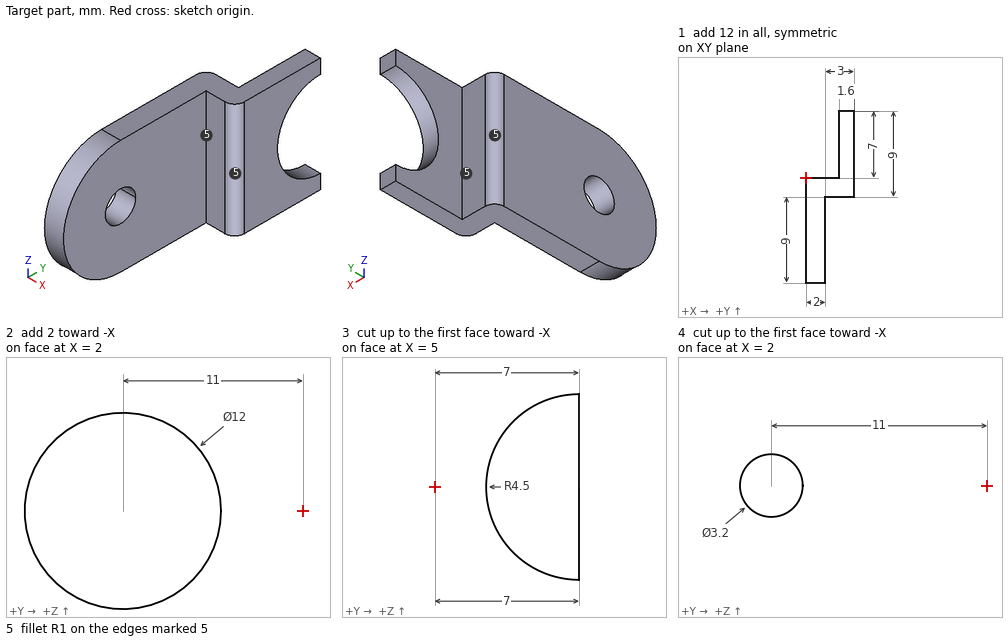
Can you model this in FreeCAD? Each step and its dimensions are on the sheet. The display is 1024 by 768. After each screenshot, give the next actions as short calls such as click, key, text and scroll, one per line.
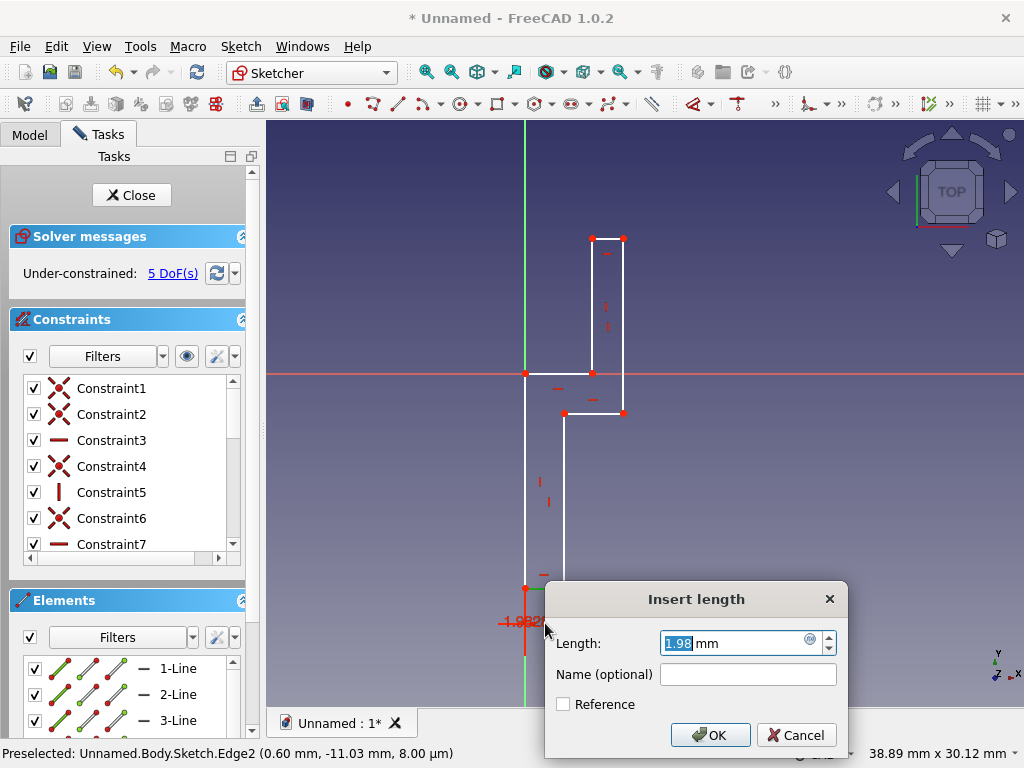
text(2)
key(Return)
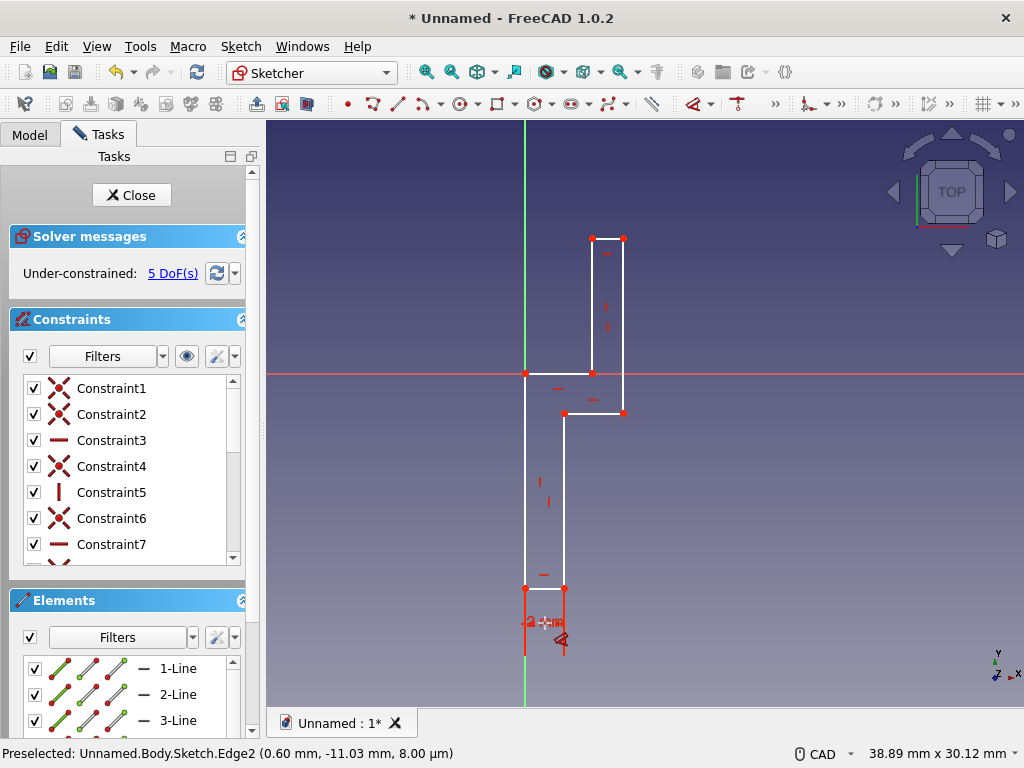
click(564, 536)
click(598, 501)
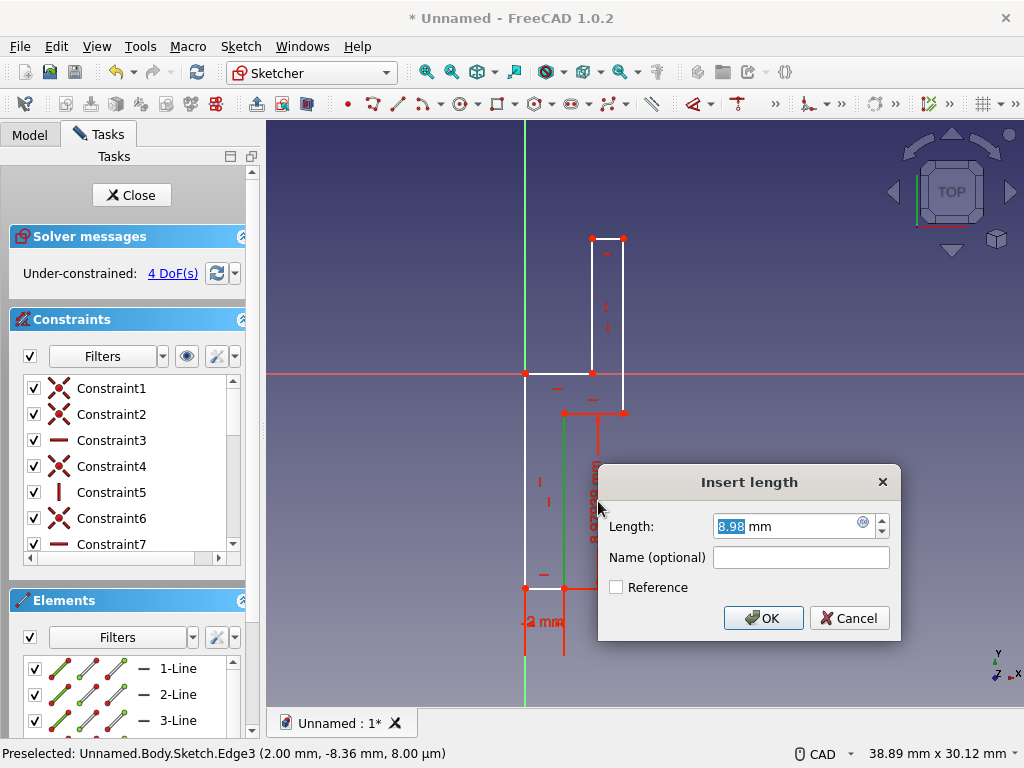
text(9)
key(Return)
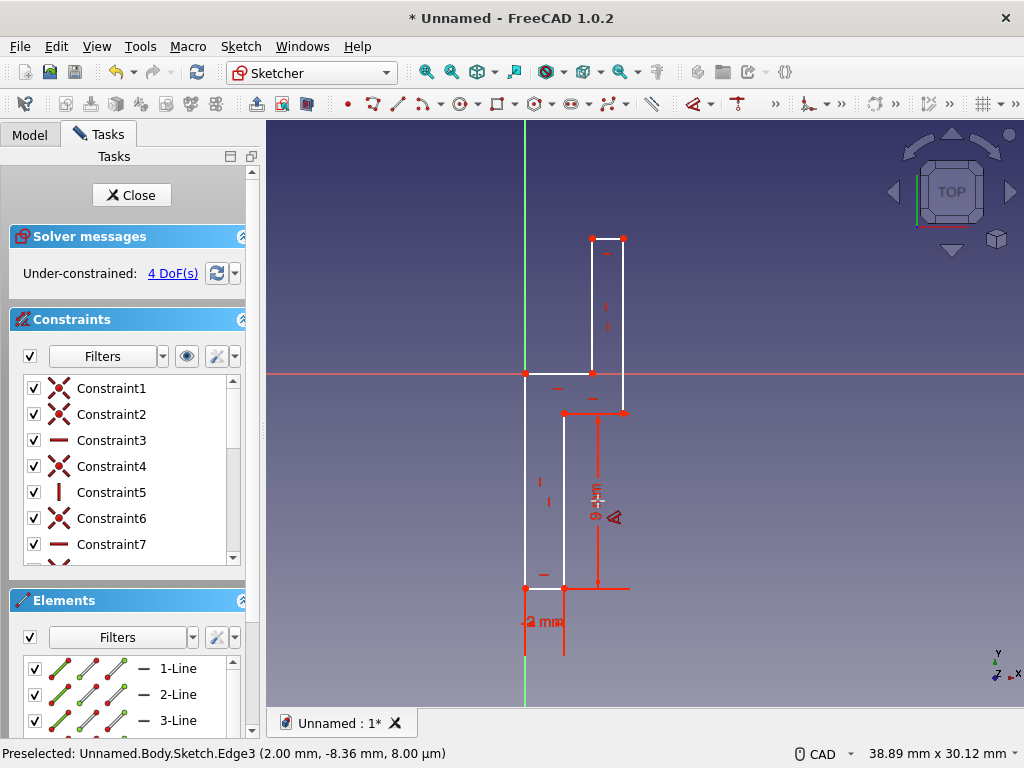
click(582, 414)
click(594, 448)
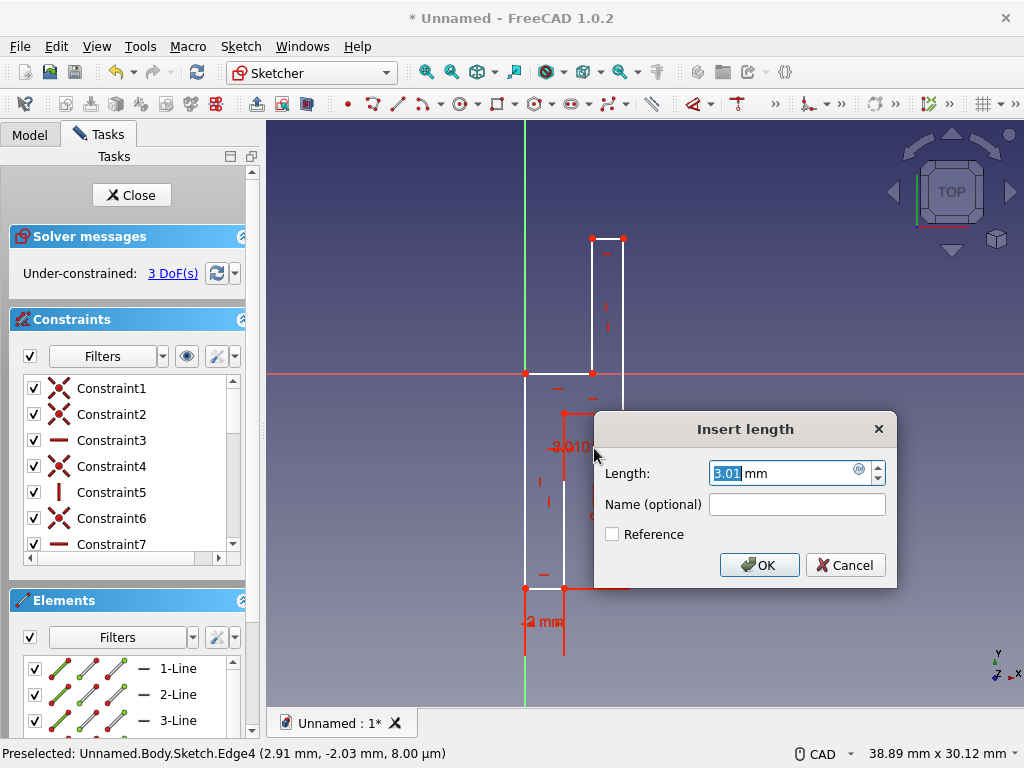
text(3)
key(Return)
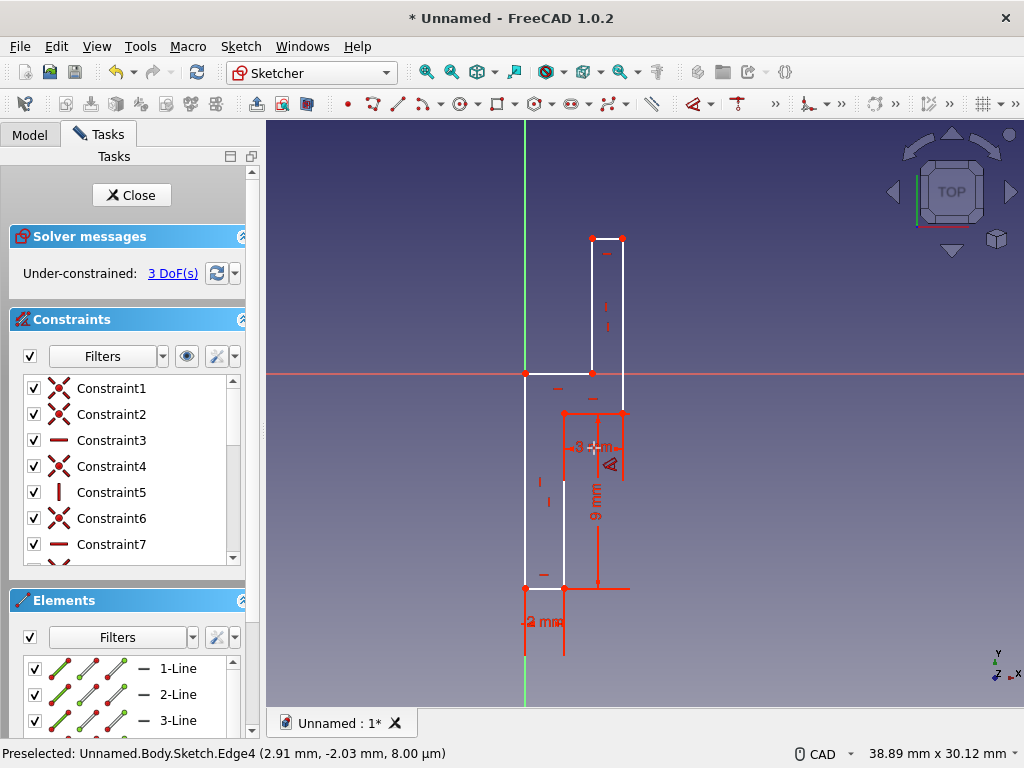
click(623, 361)
click(657, 326)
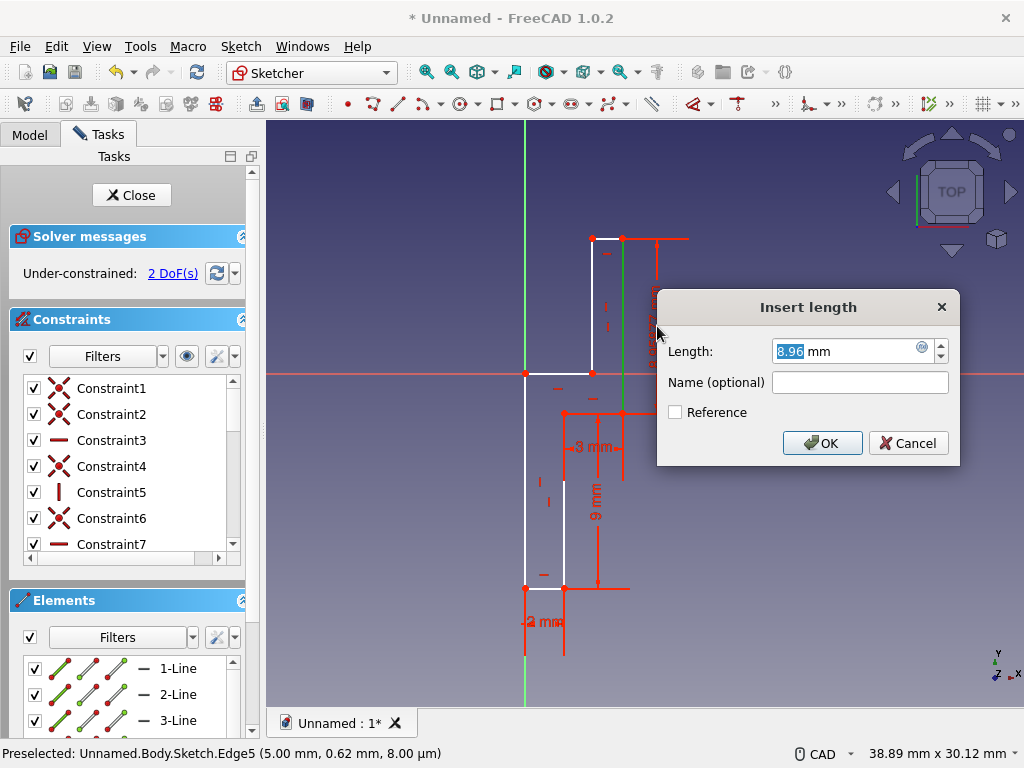
text(9)
key(Return)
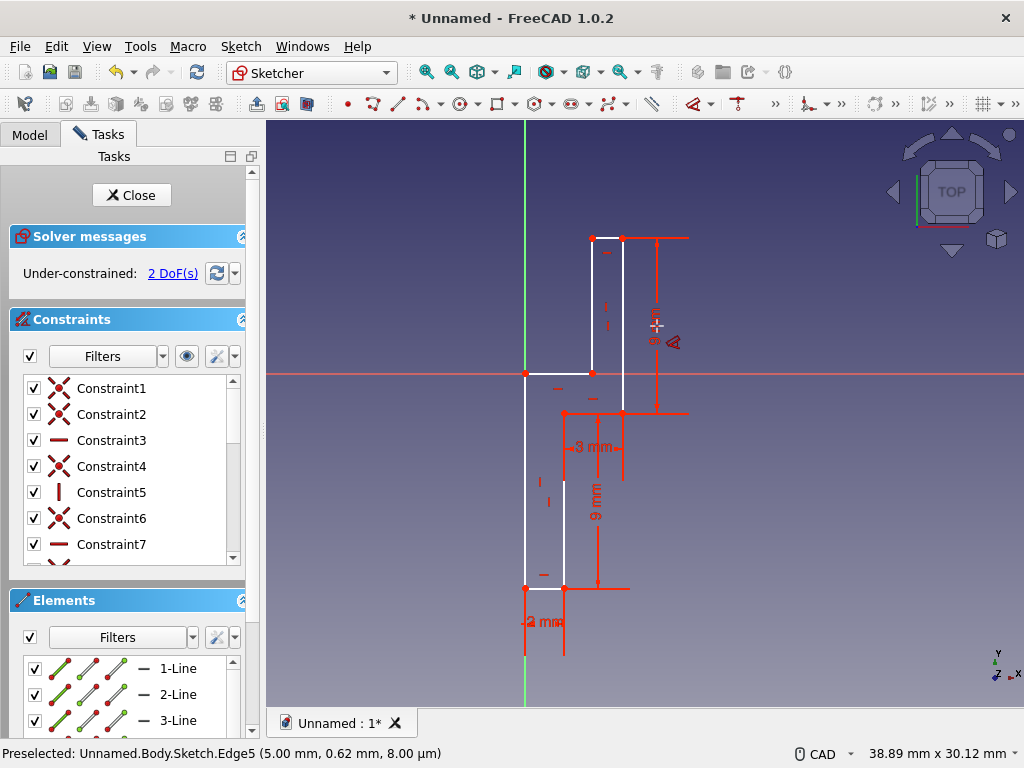
click(592, 279)
click(558, 306)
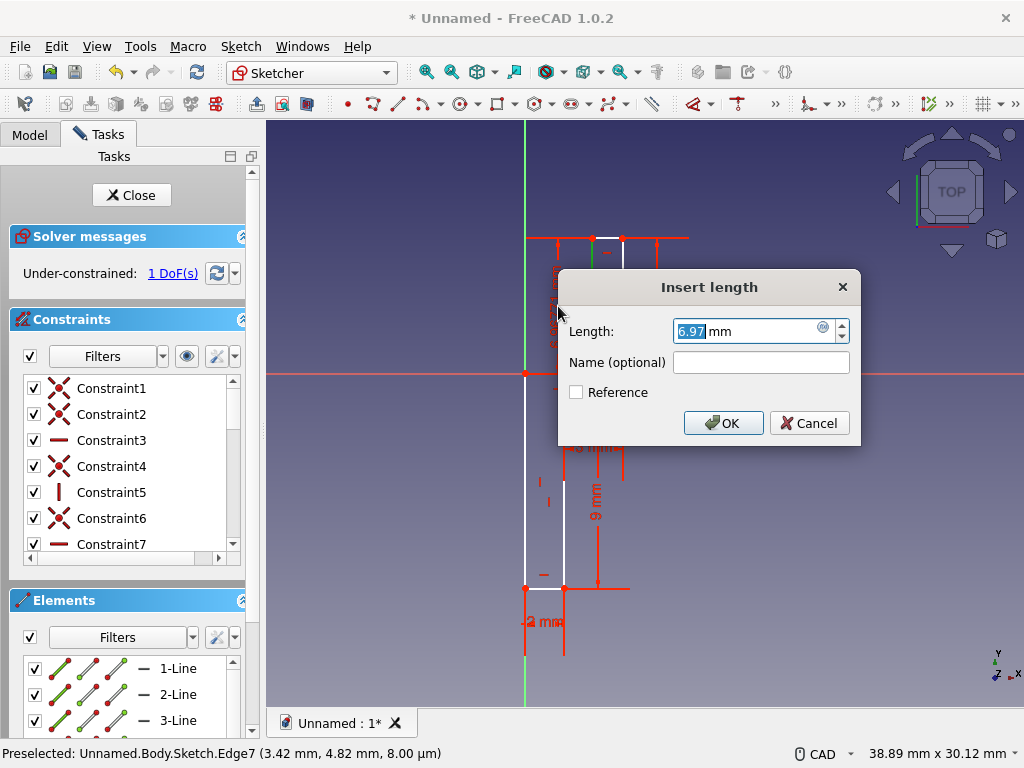
text(7)
key(Return)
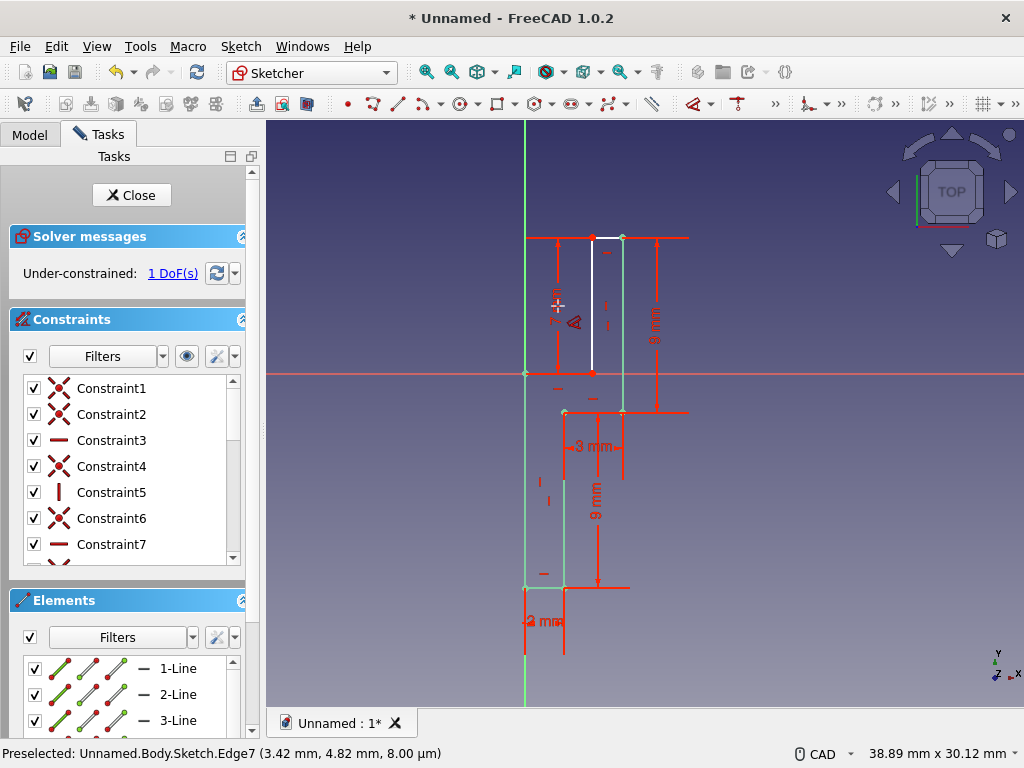
scroll(614, 238, up, 3)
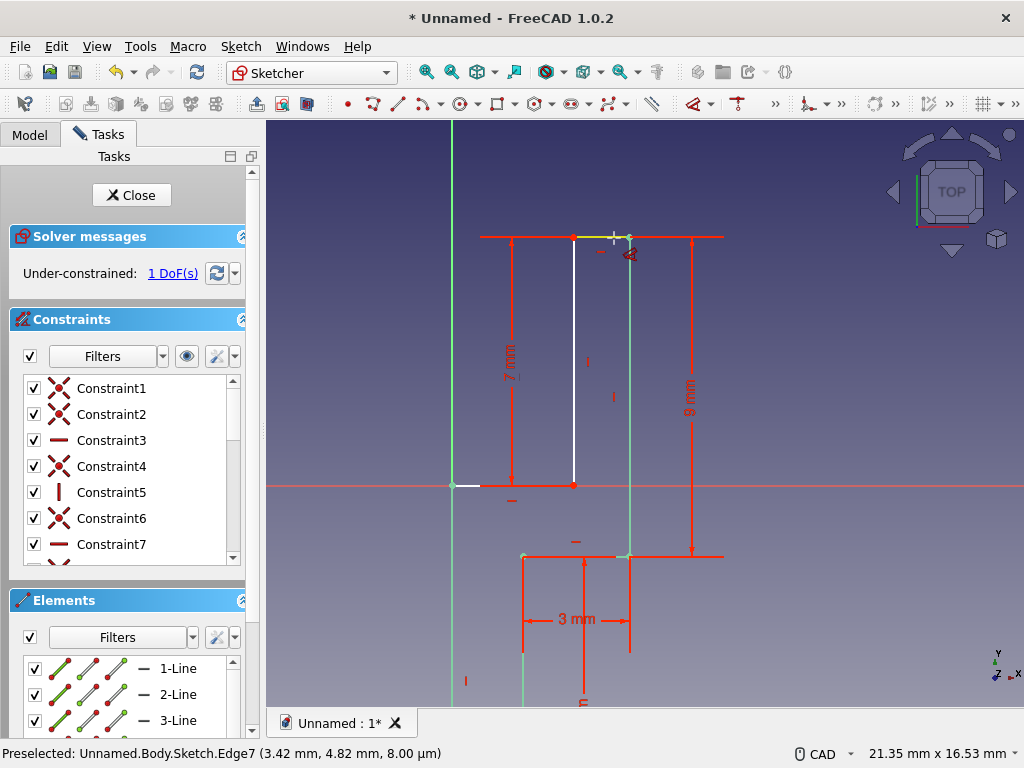
click(613, 237)
click(602, 203)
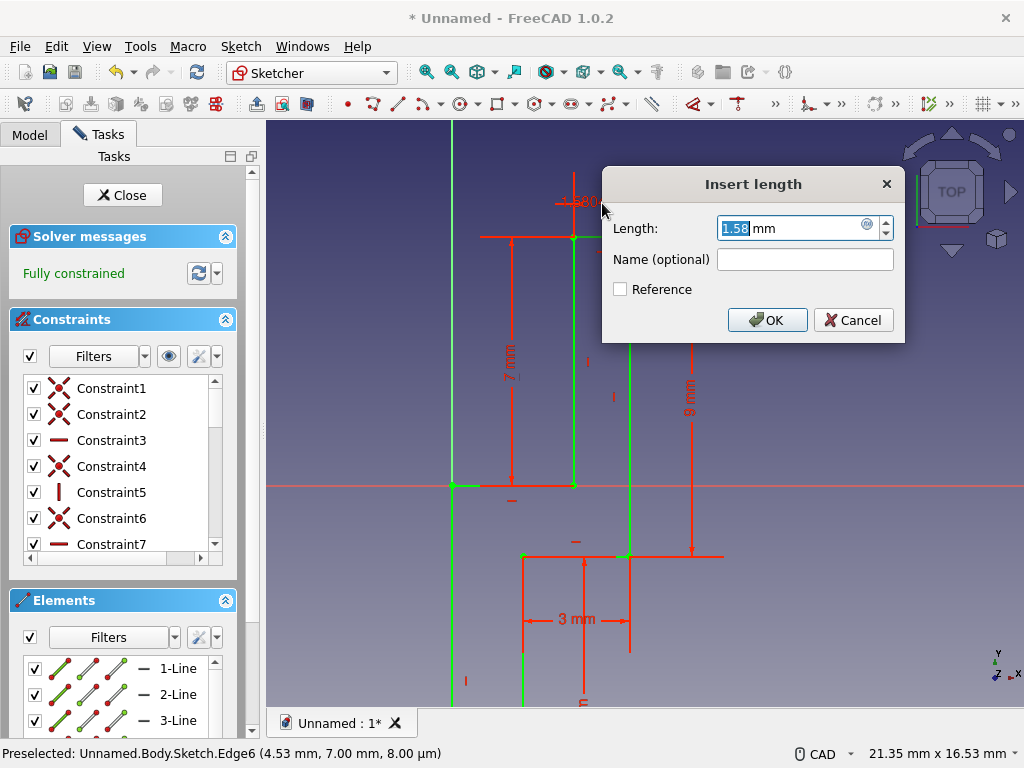
text(1.6)
key(Return)
key(Escape)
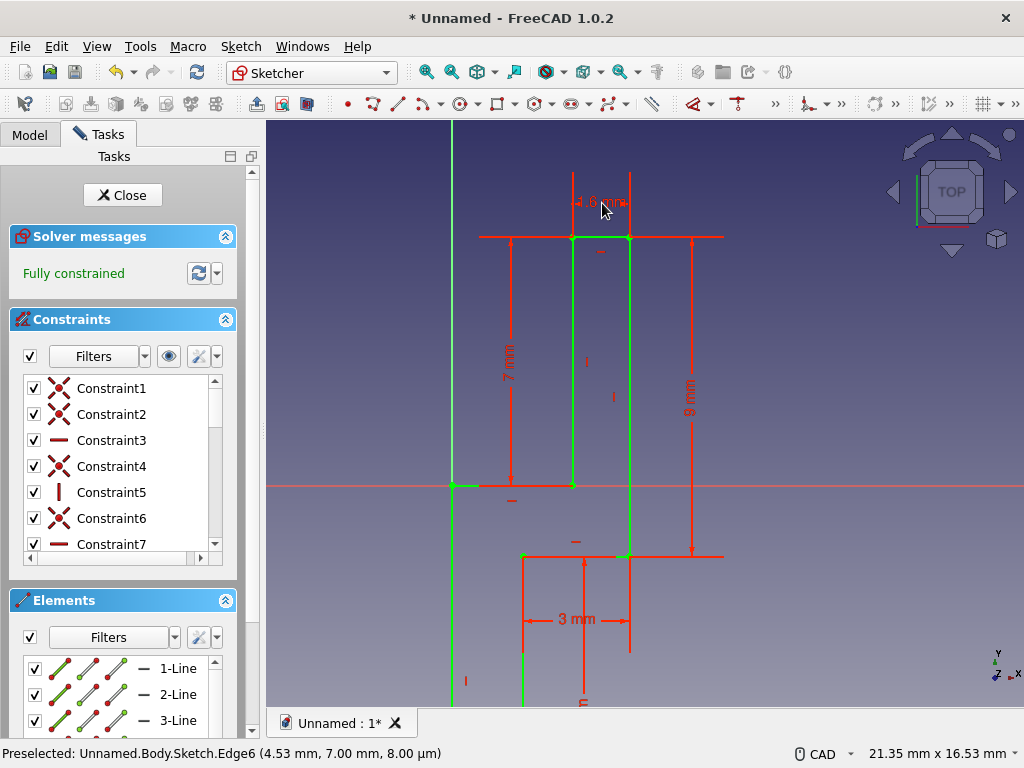
click(123, 195)